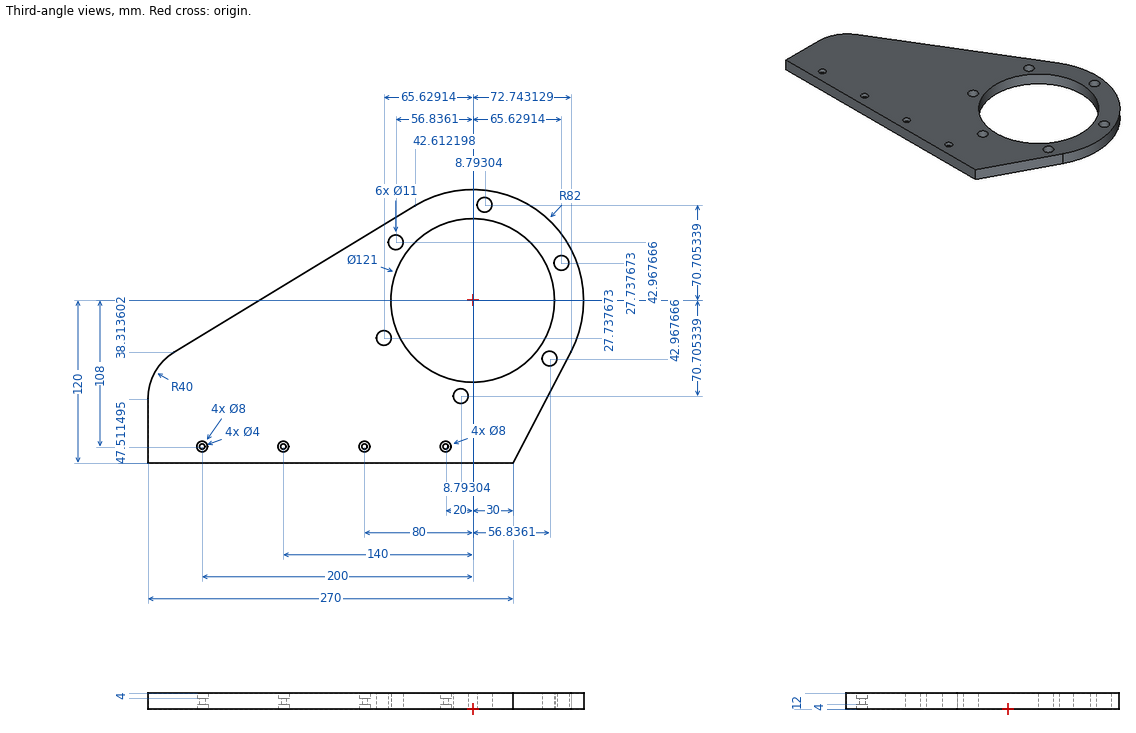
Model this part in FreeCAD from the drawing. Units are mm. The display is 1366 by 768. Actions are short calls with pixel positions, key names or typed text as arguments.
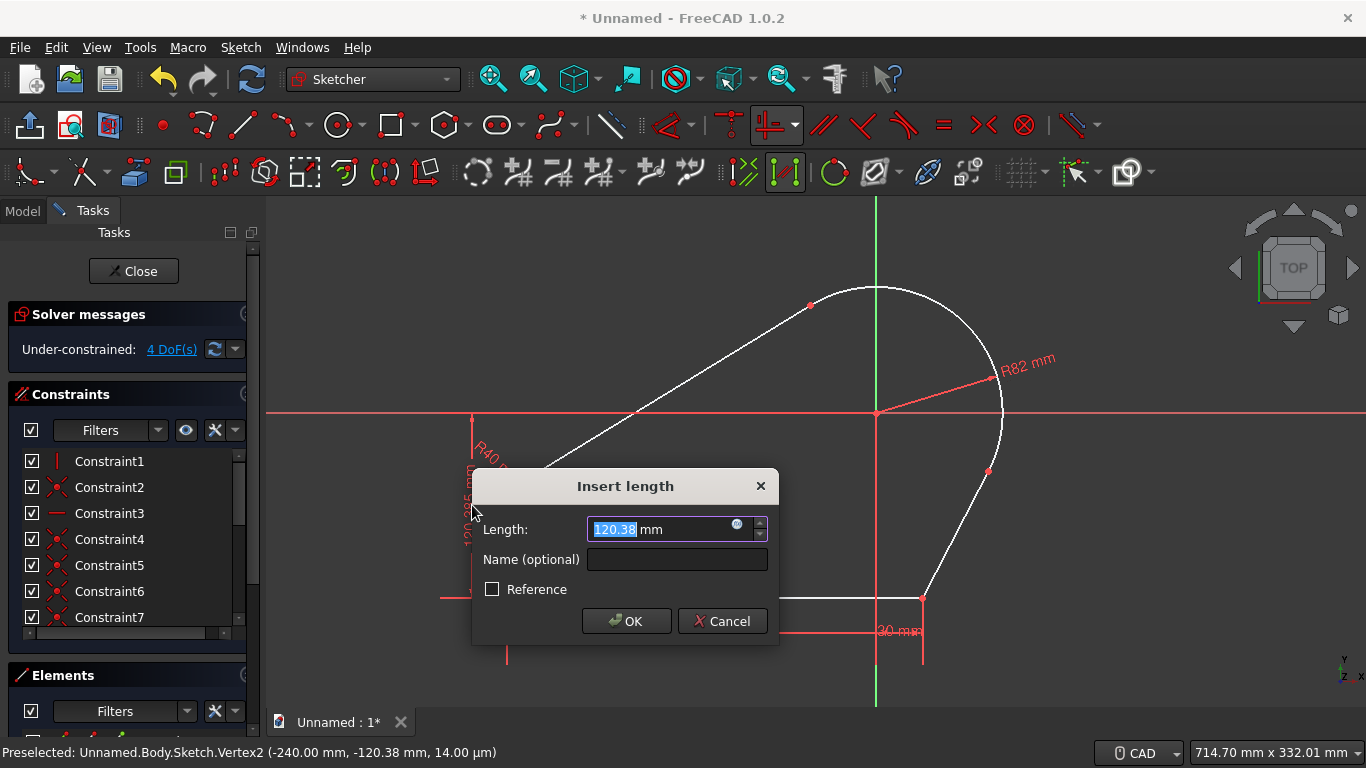
text(120)
key(Return)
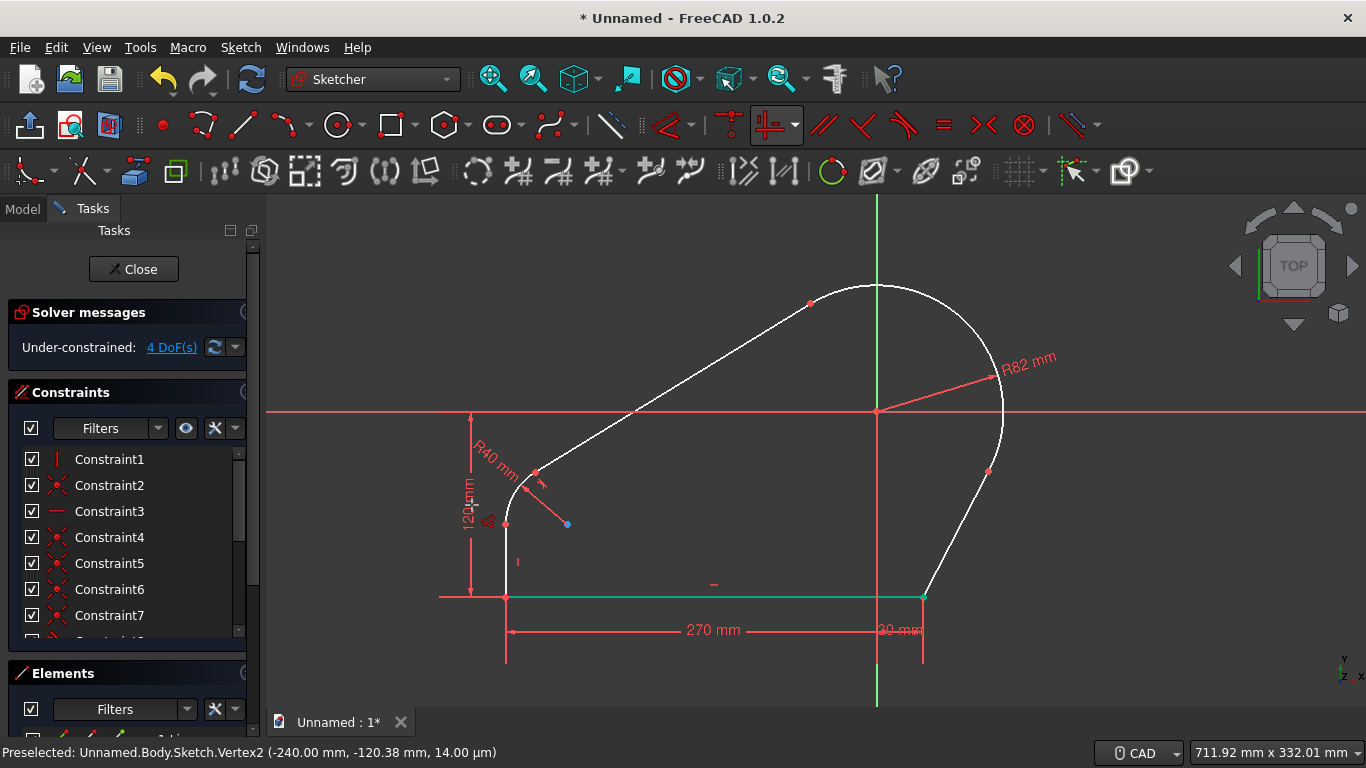
click(506, 547)
click(472, 561)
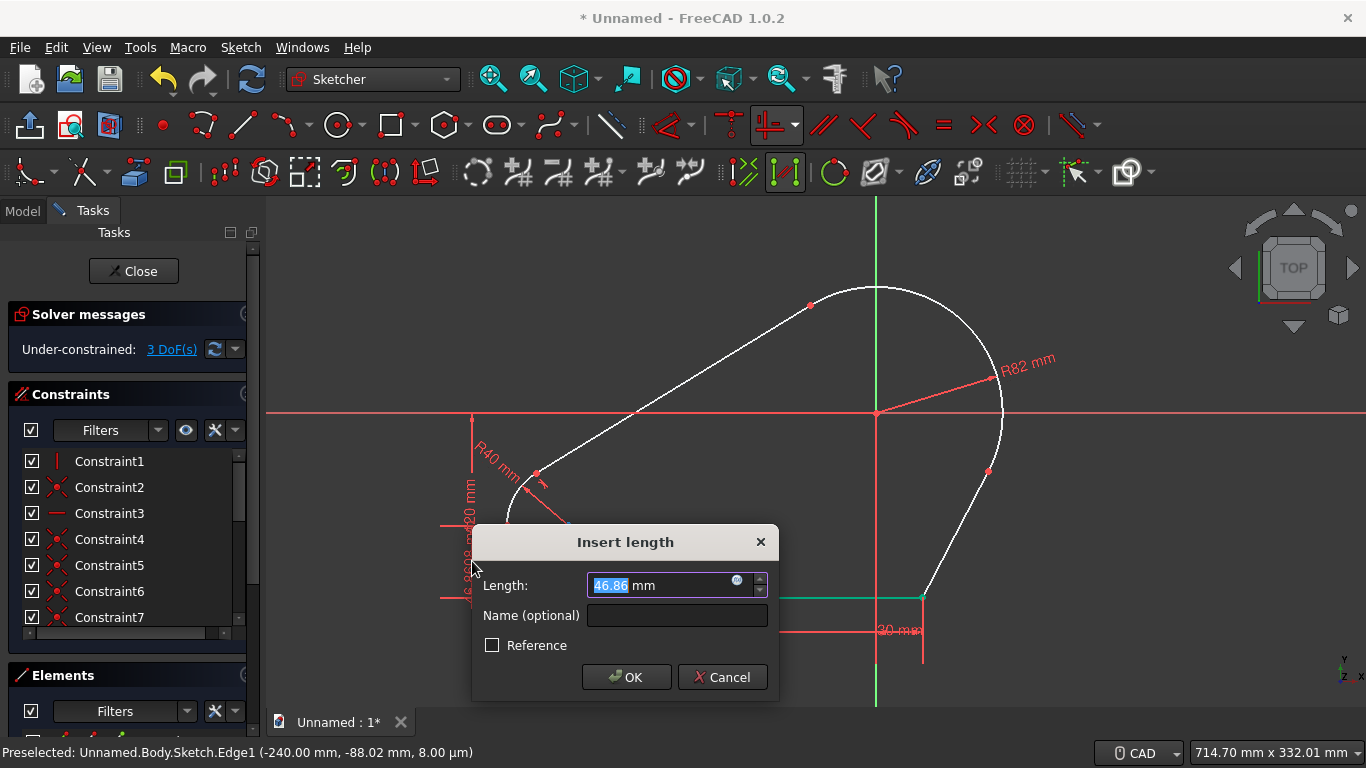
text(47.511495)
key(Return)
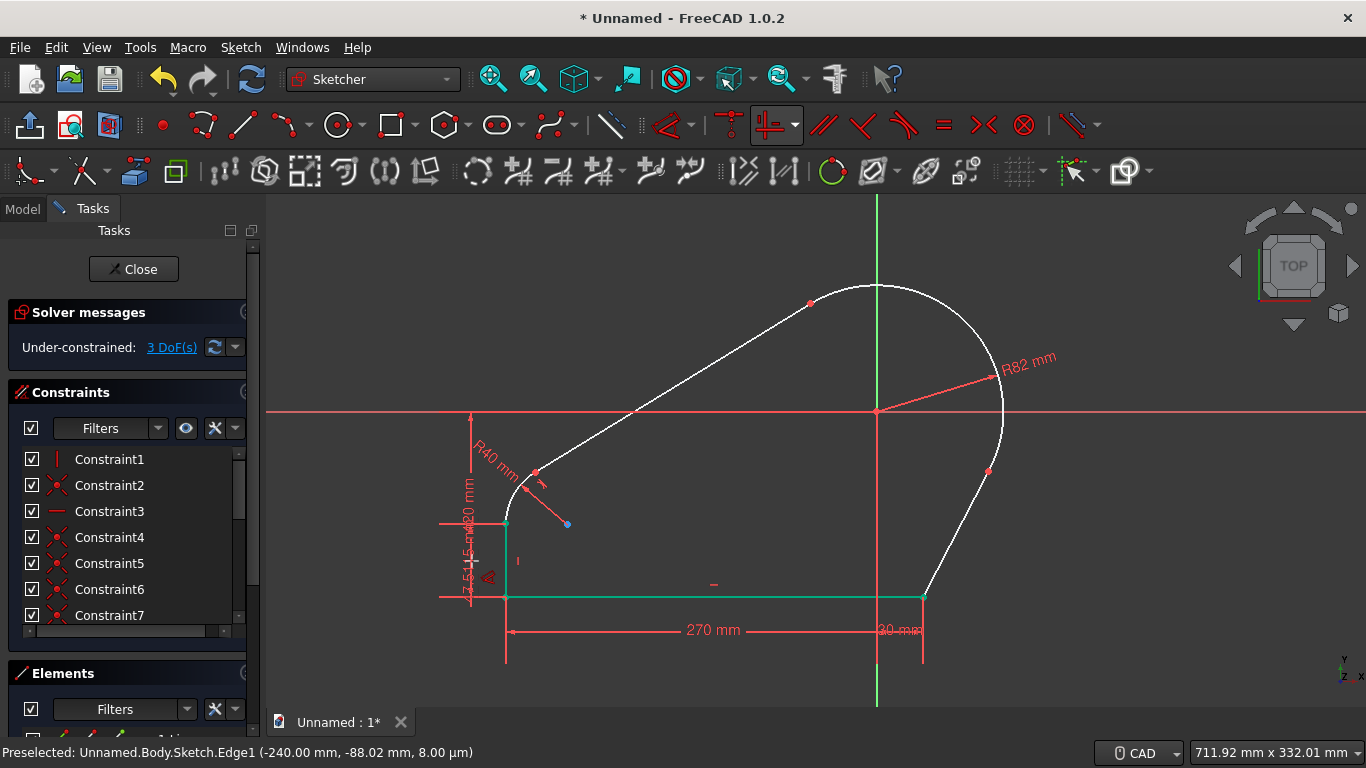
click(989, 471)
click(933, 378)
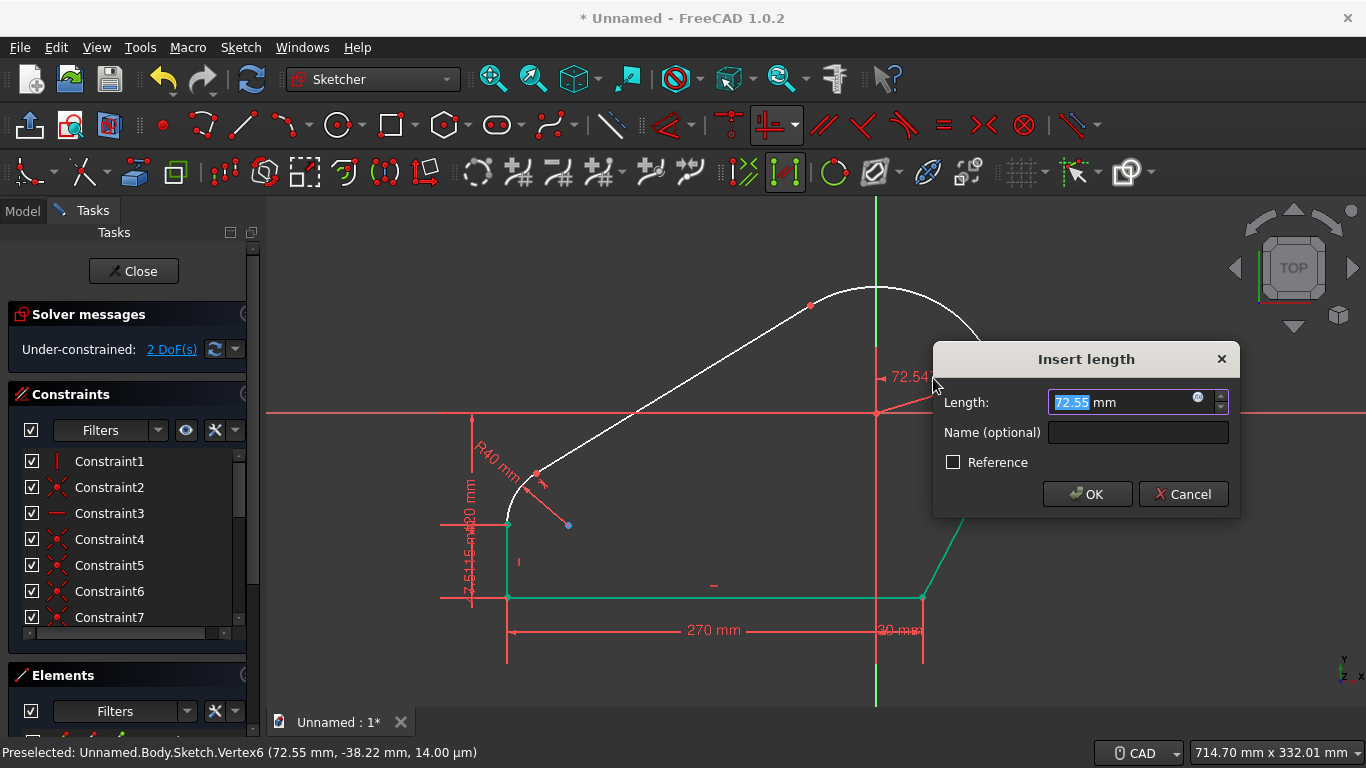
text(72.743129)
key(Return)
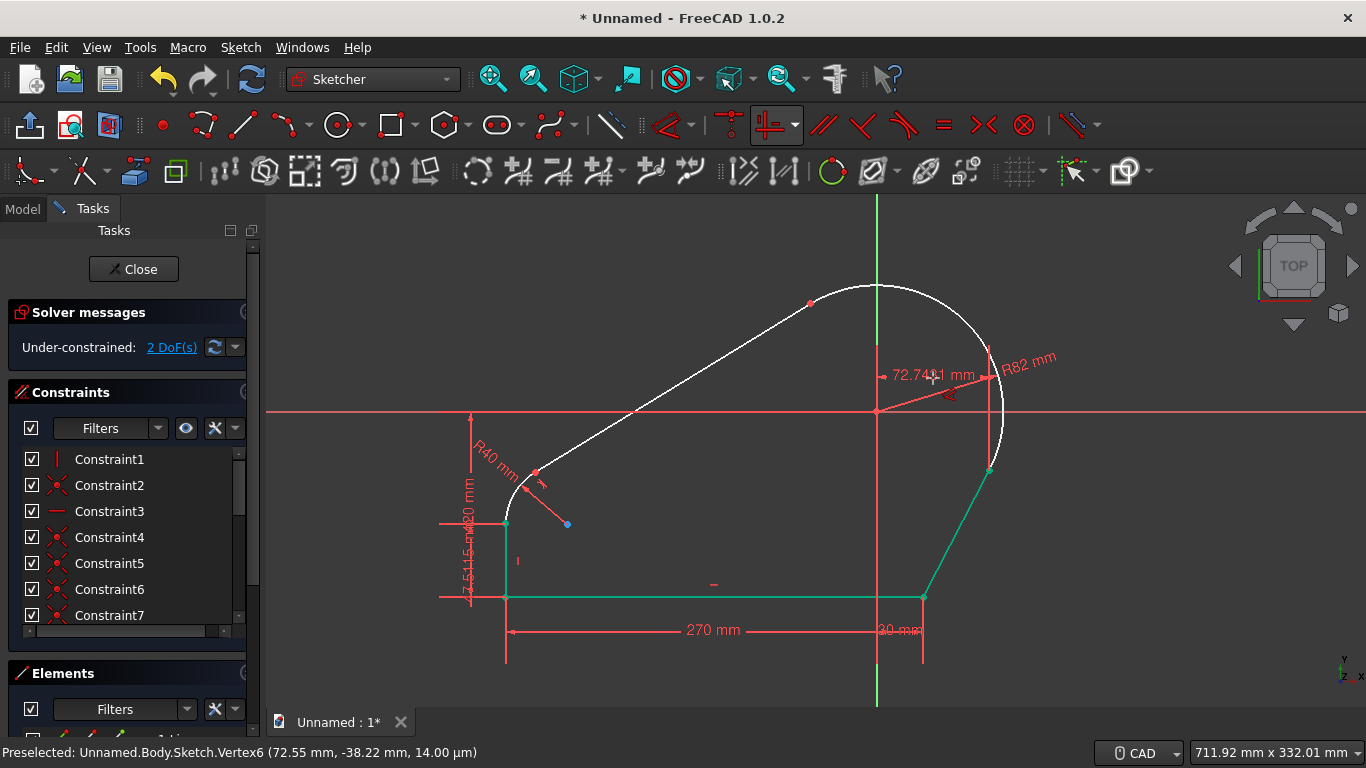
click(810, 304)
click(844, 270)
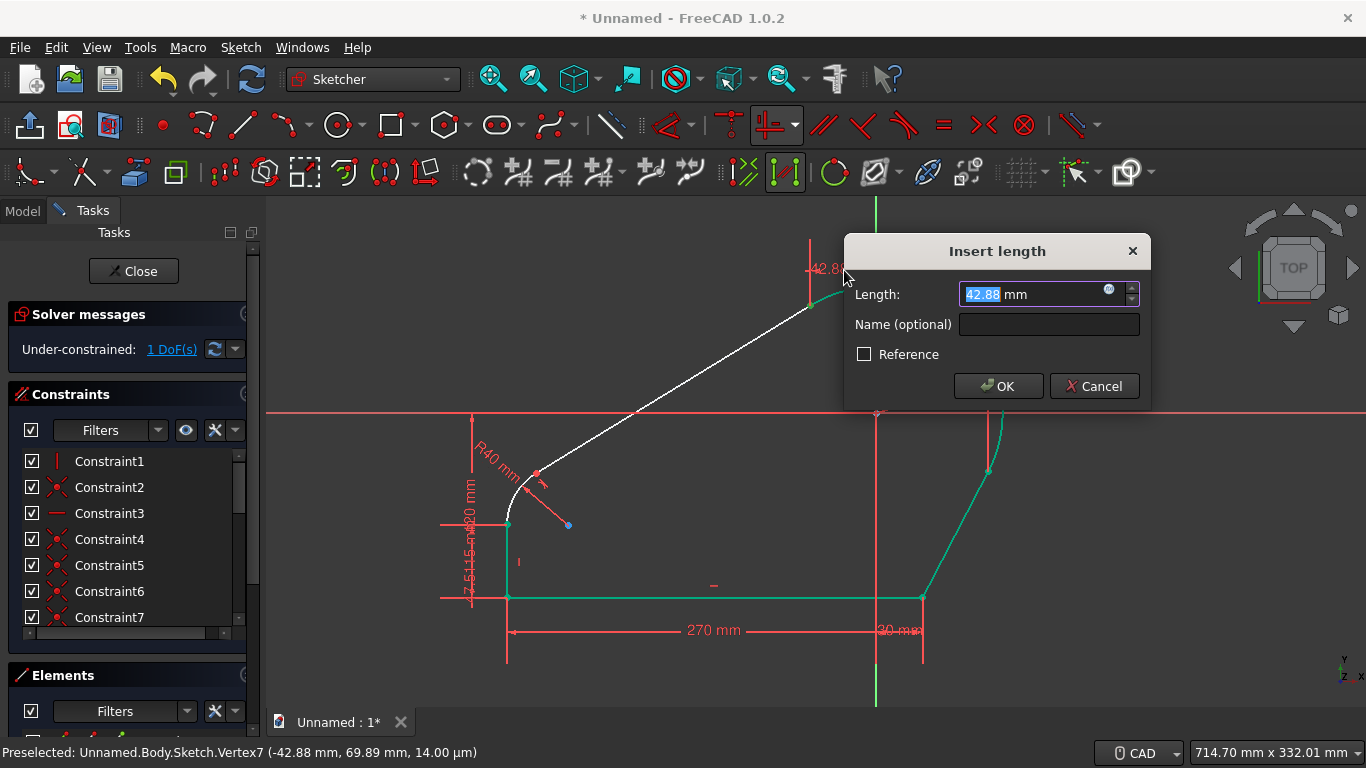
text(42.612198)
key(Return)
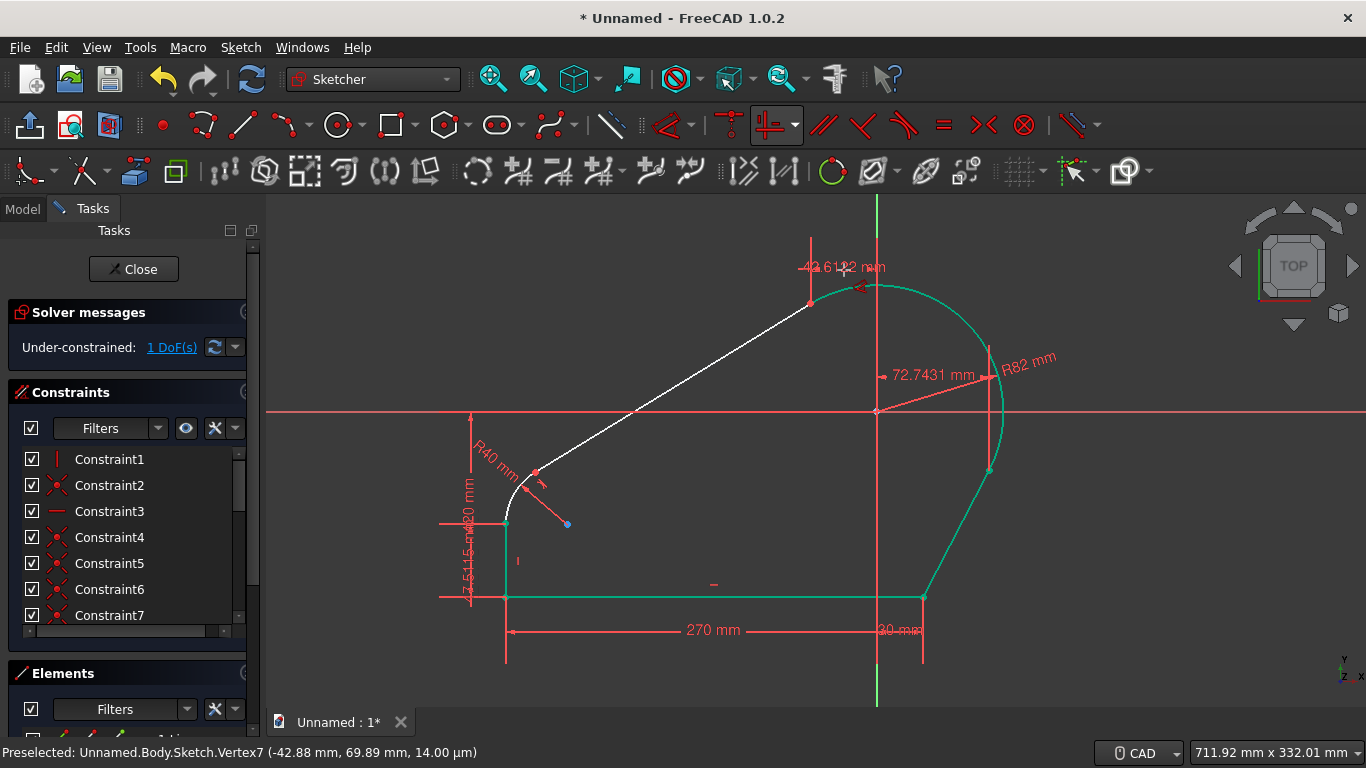
click(535, 472)
click(501, 442)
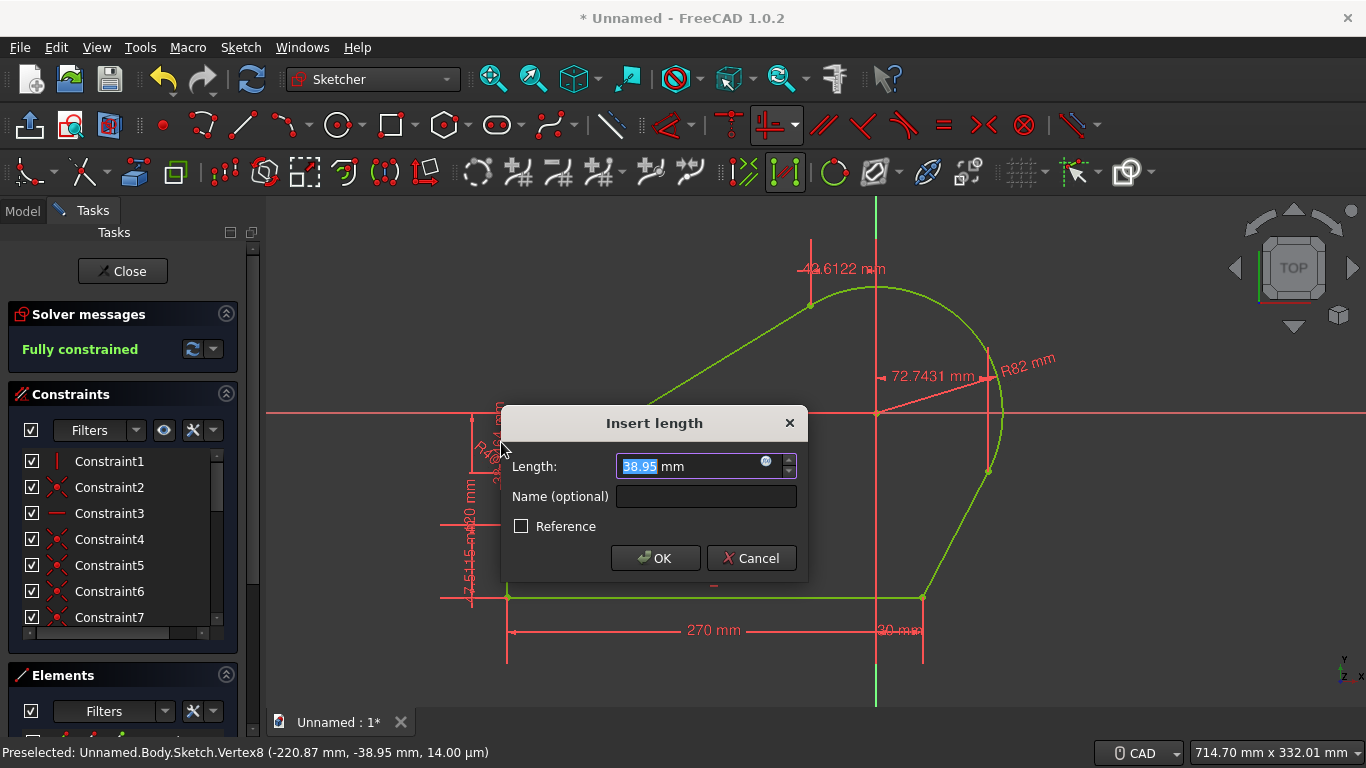
text(38.313602)
key(Return)
key(Escape)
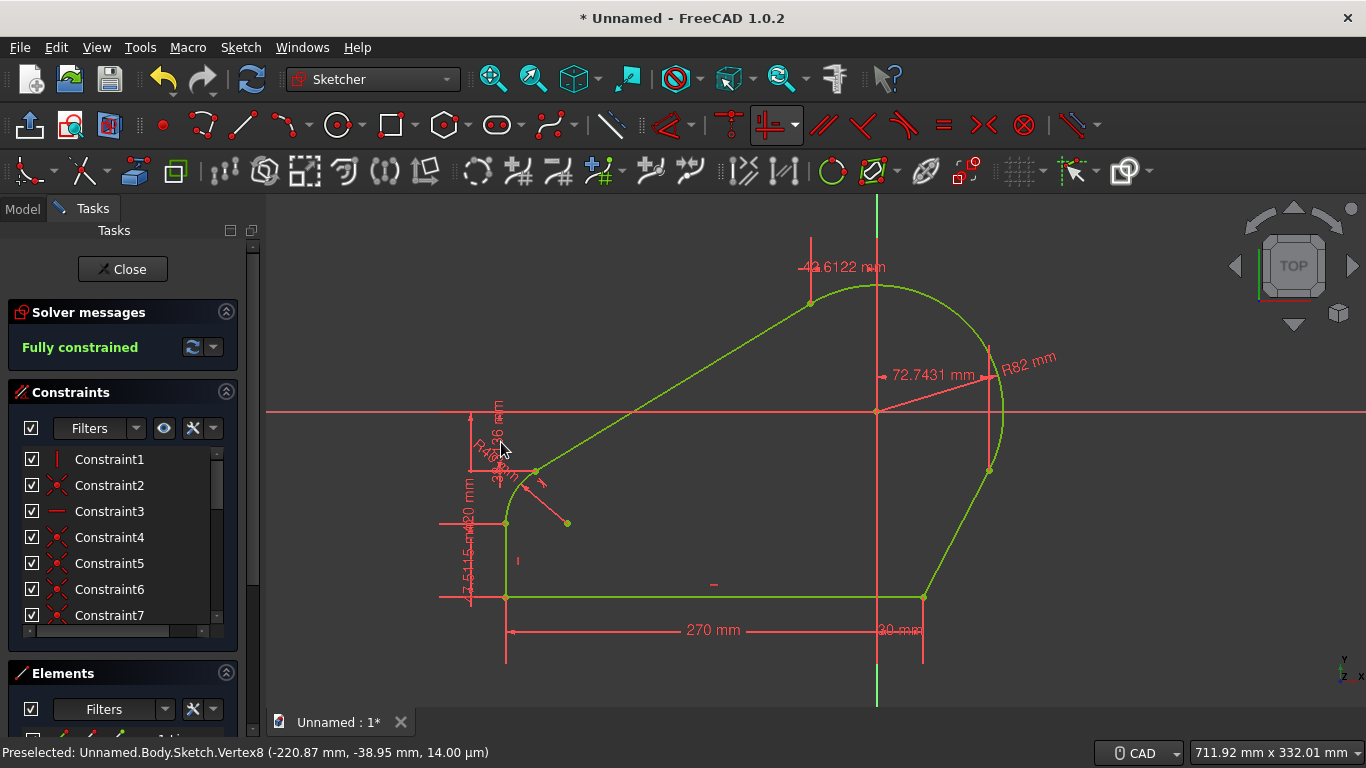
click(123, 269)